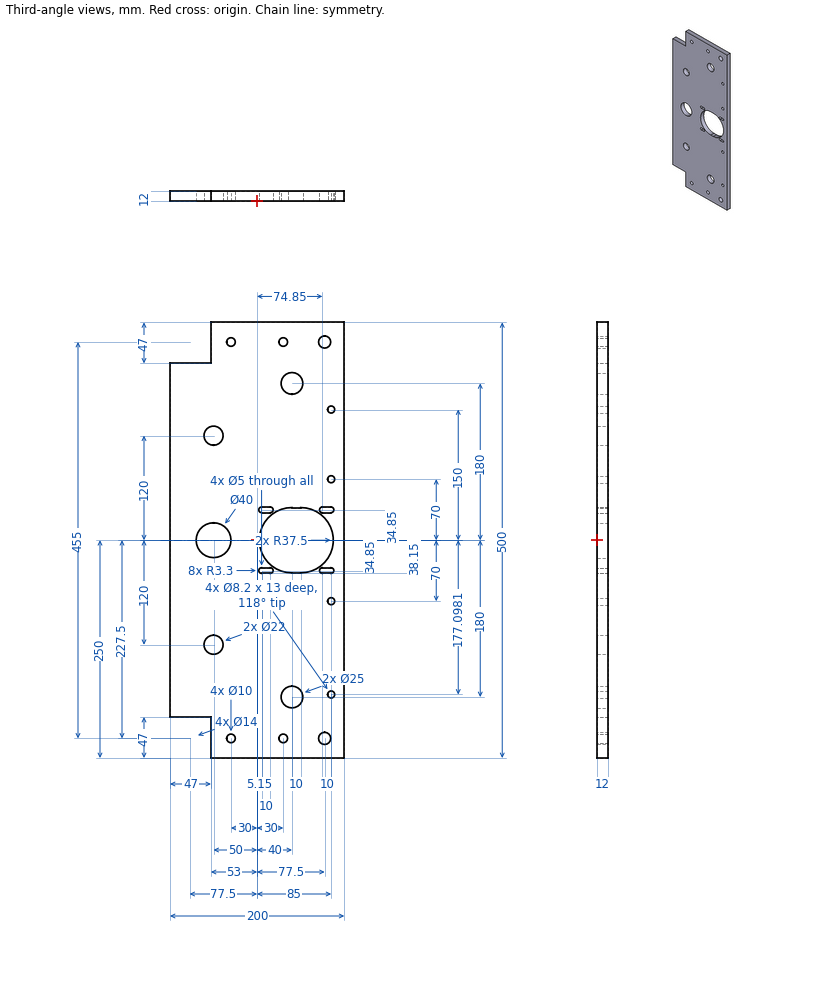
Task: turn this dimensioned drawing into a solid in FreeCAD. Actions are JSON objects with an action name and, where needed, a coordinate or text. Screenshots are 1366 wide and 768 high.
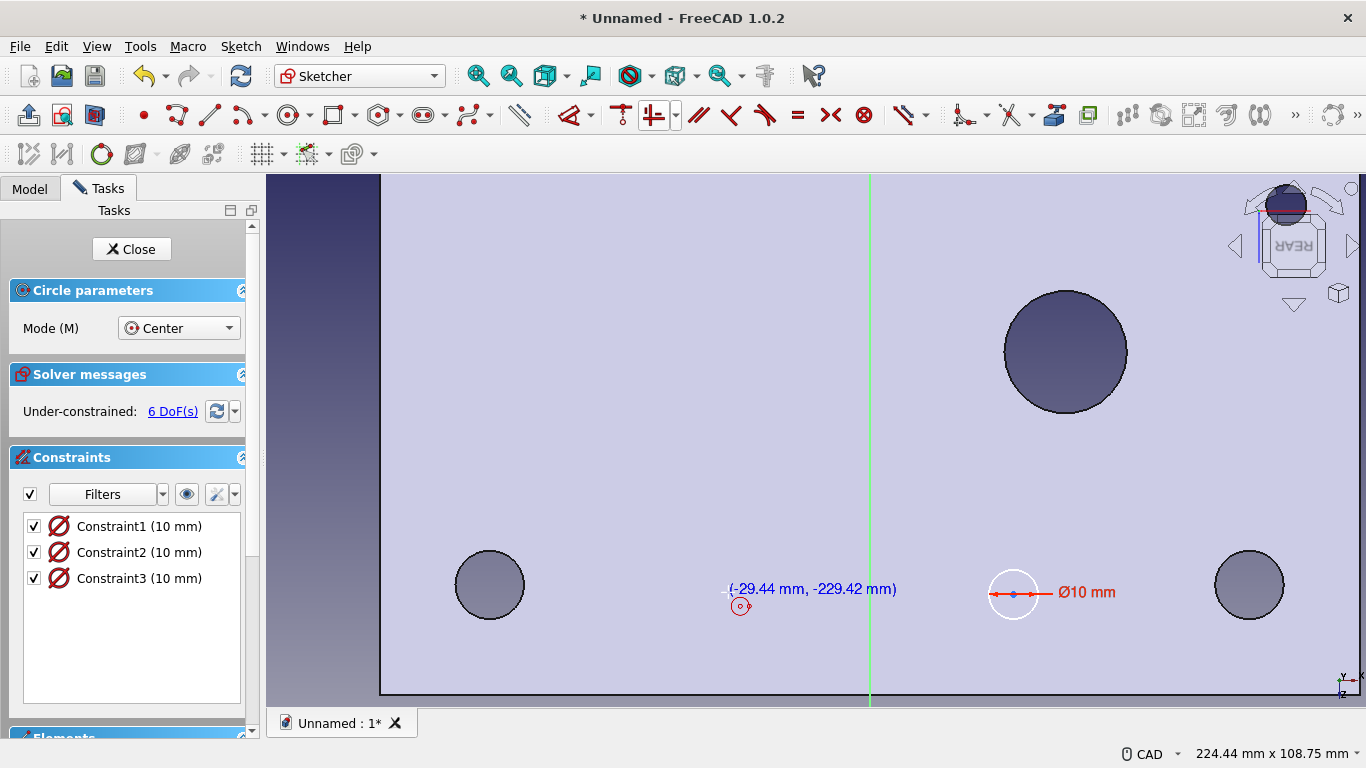
{"action": "scroll", "coordinate": [728, 592], "scroll_direction": "down", "scroll_amount": 10}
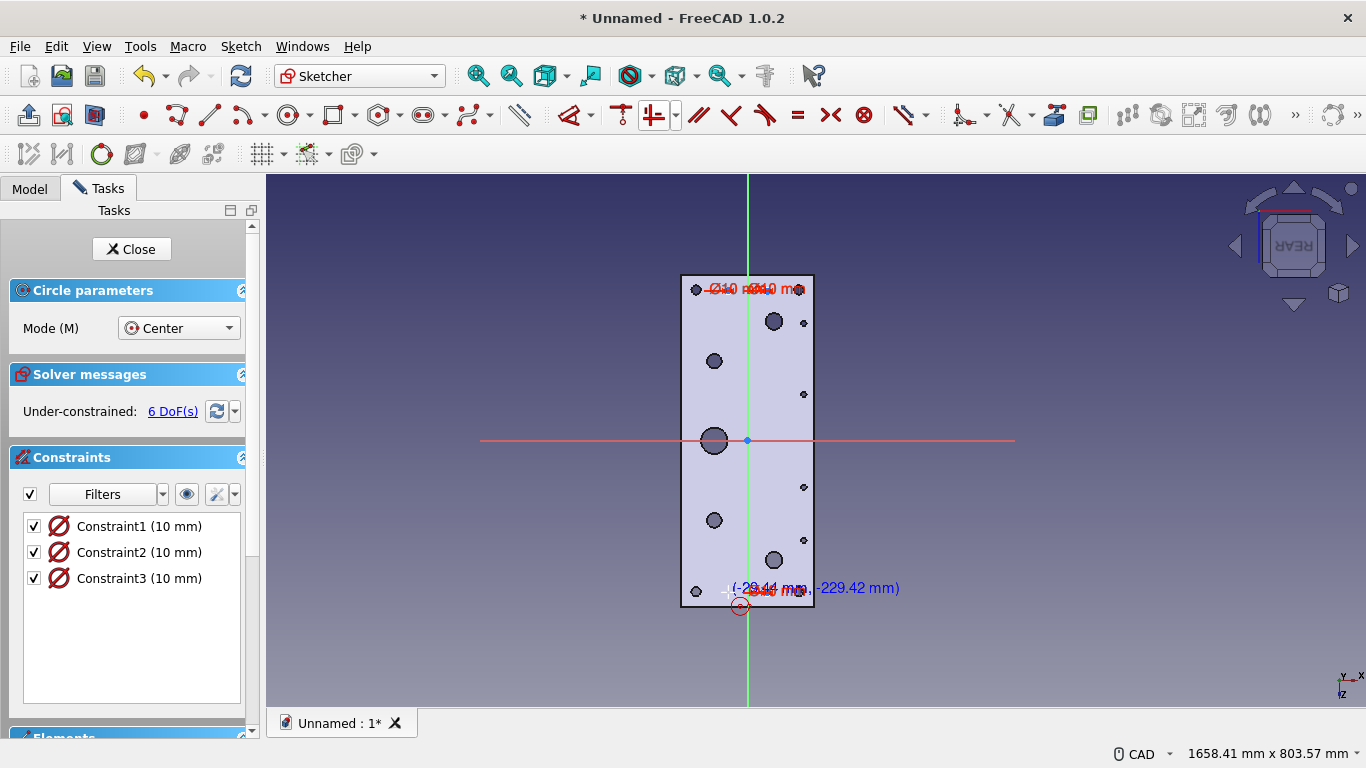
{"action": "left_click", "coordinate": [728, 592]}
{"action": "mouse_move", "coordinate": [730, 589]}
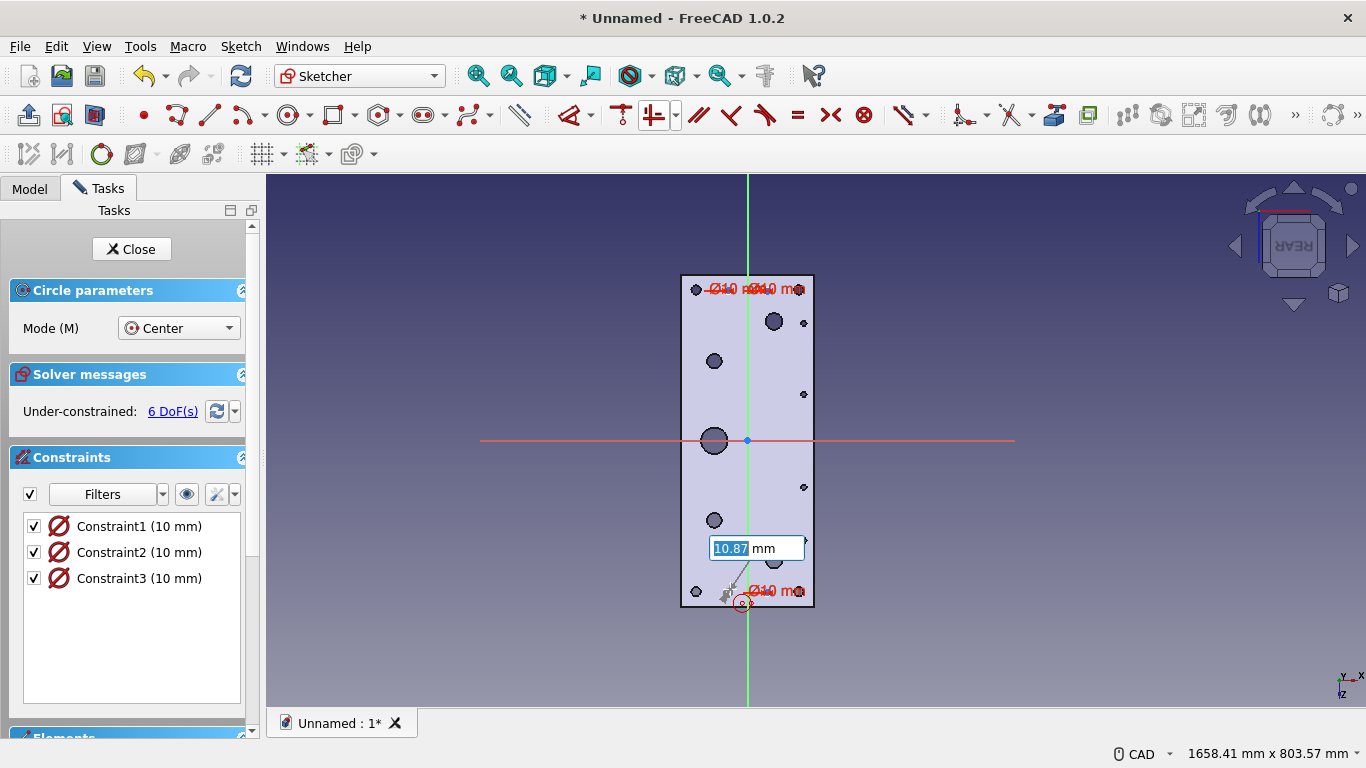
{"action": "type", "text": "10"}
{"action": "key", "text": "Return"}
{"action": "key", "text": "Escape"}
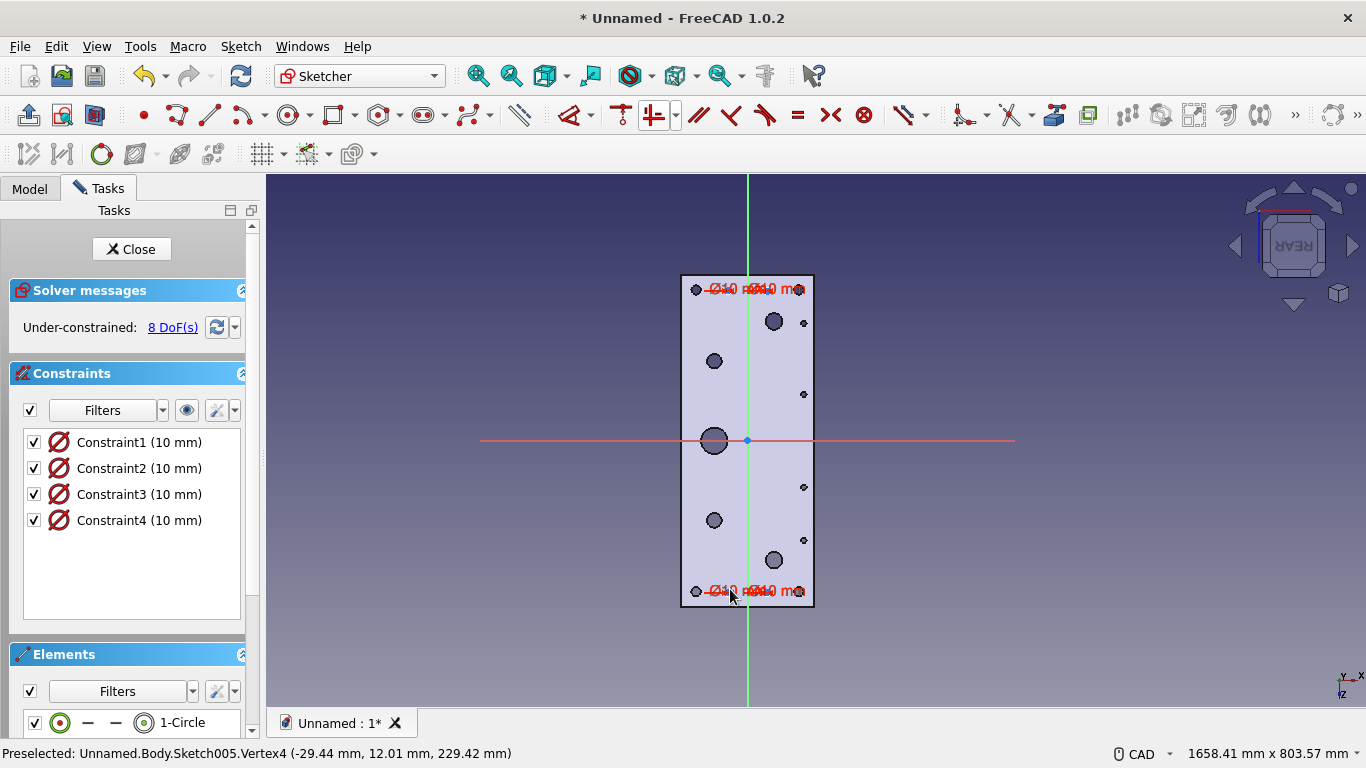
{"action": "left_click", "coordinate": [728, 291]}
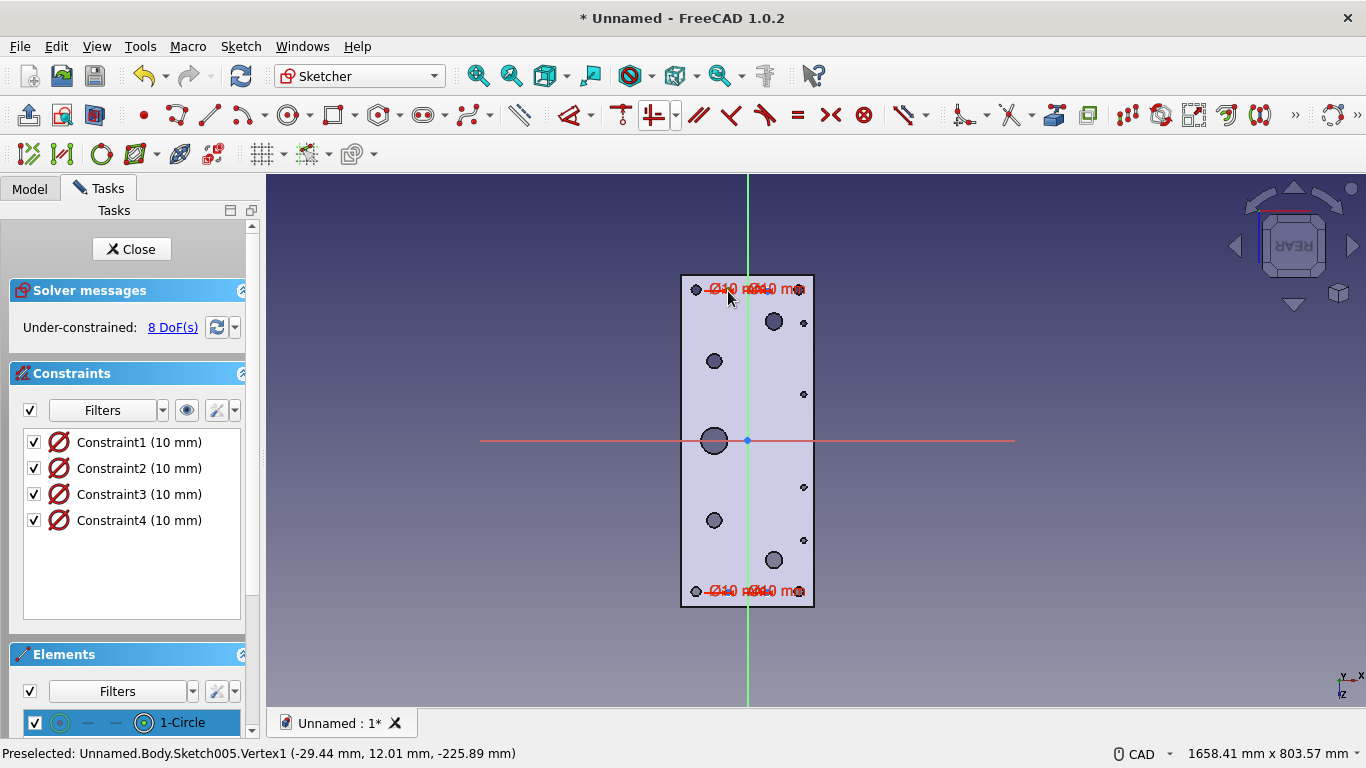
{"action": "left_click", "coordinate": [767, 291]}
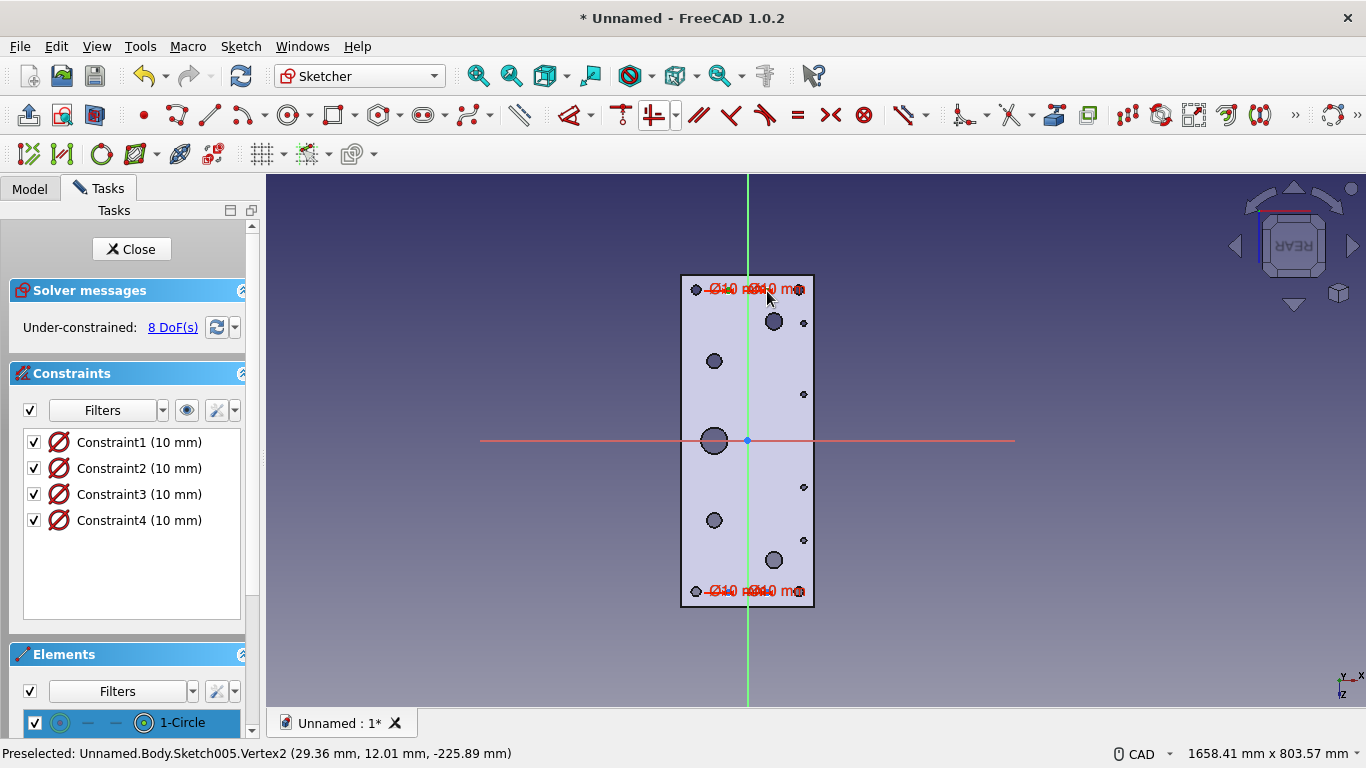
{"action": "key", "text": "h"}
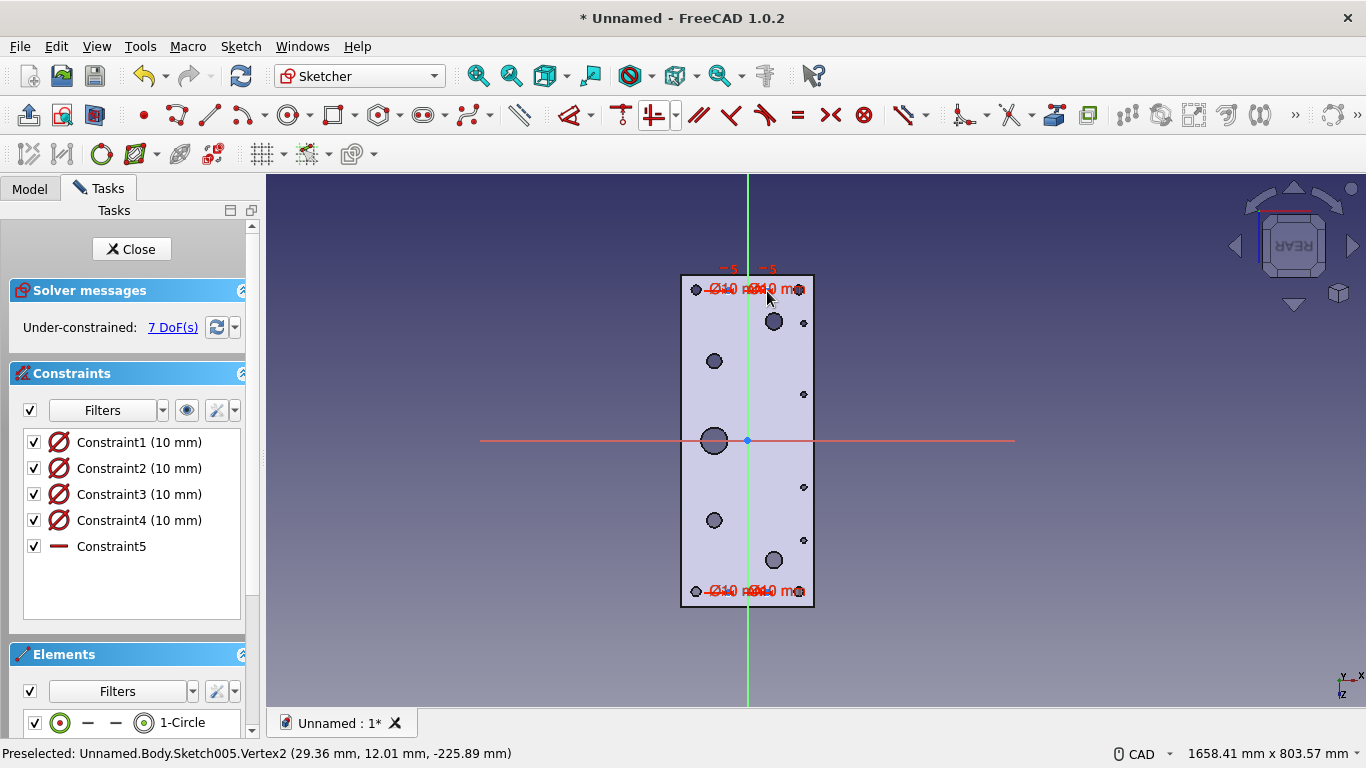
{"action": "left_click", "coordinate": [767, 291]}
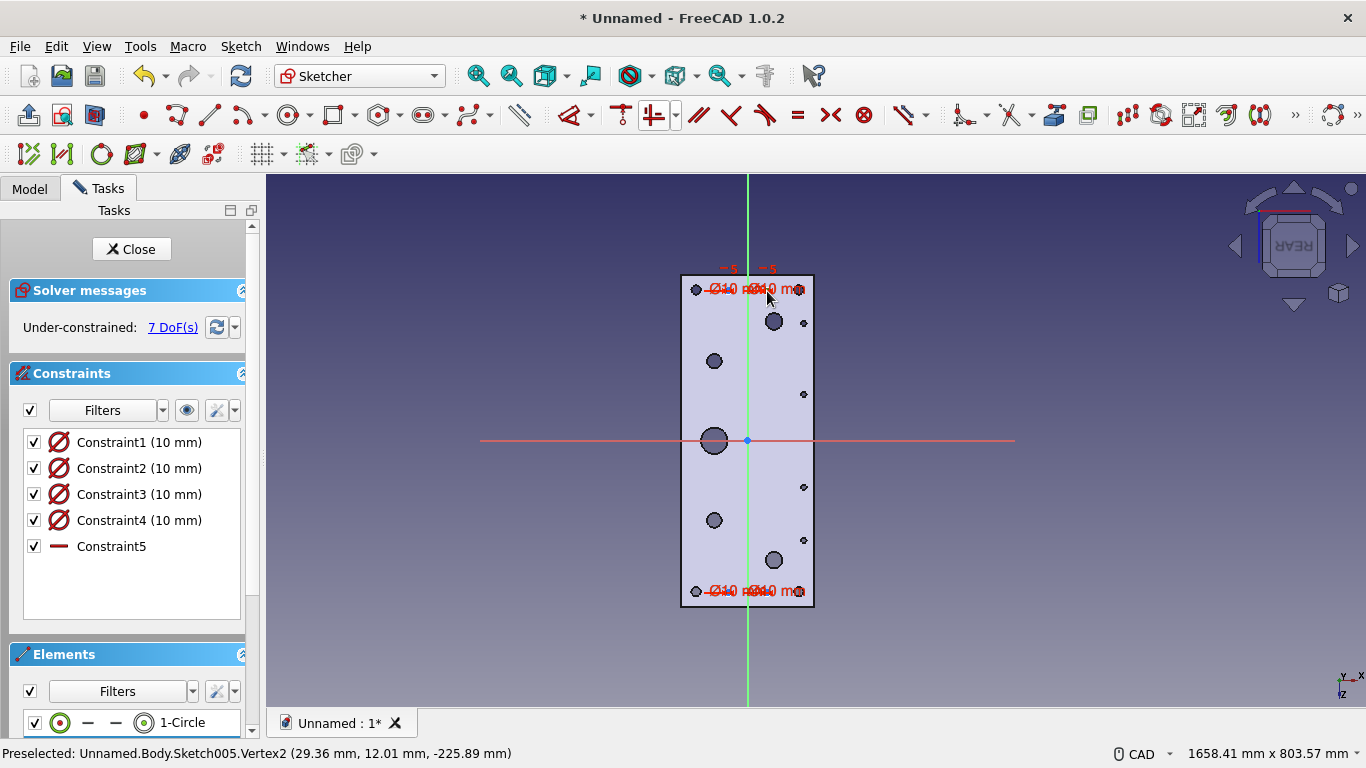
{"action": "left_click", "coordinate": [767, 593]}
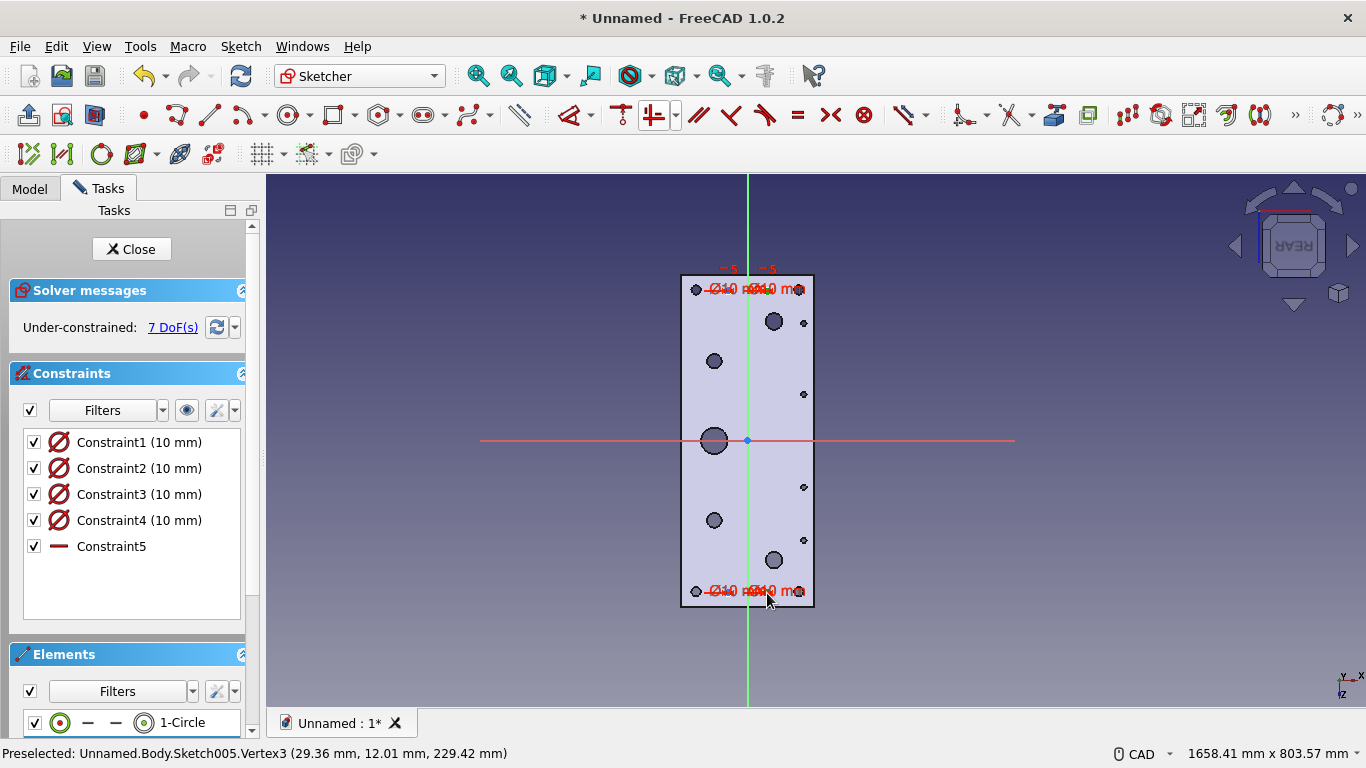
{"action": "key", "text": "v"}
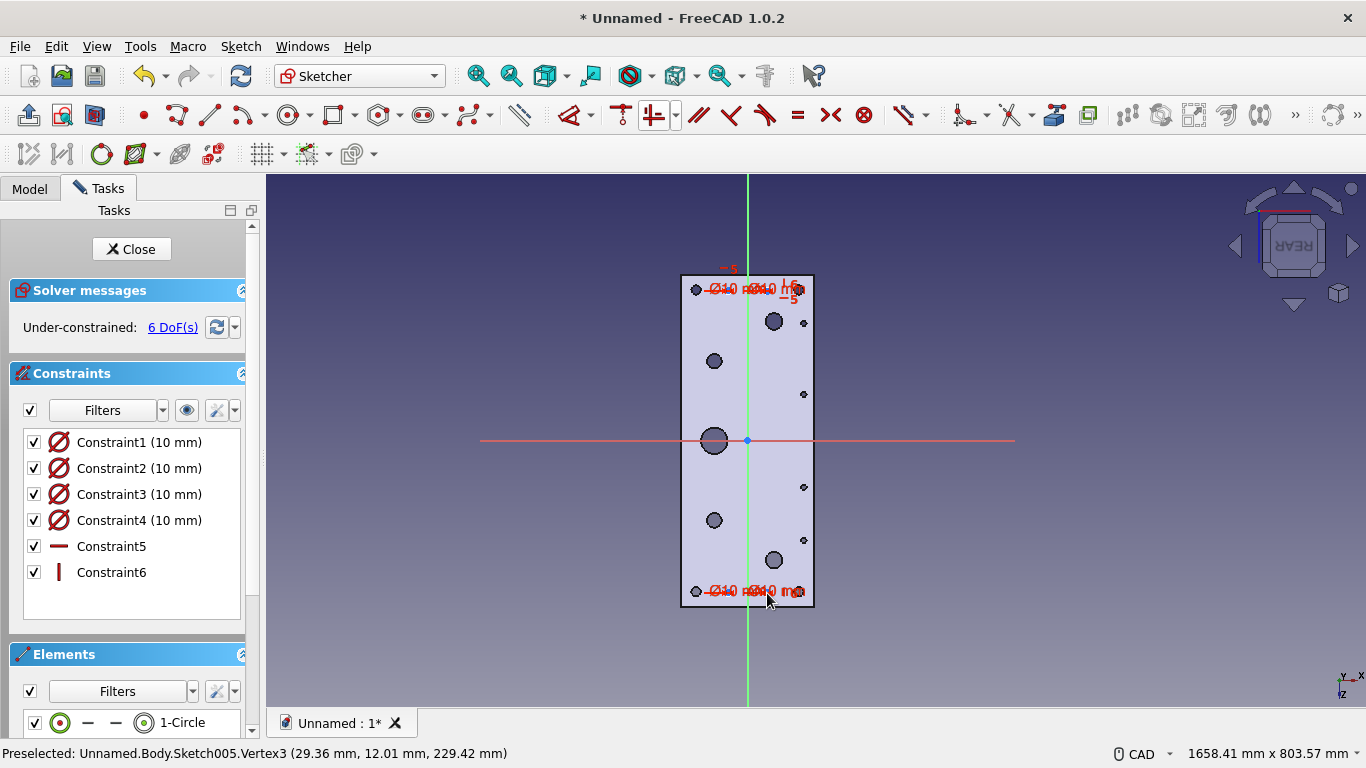
{"action": "left_click", "coordinate": [728, 291]}